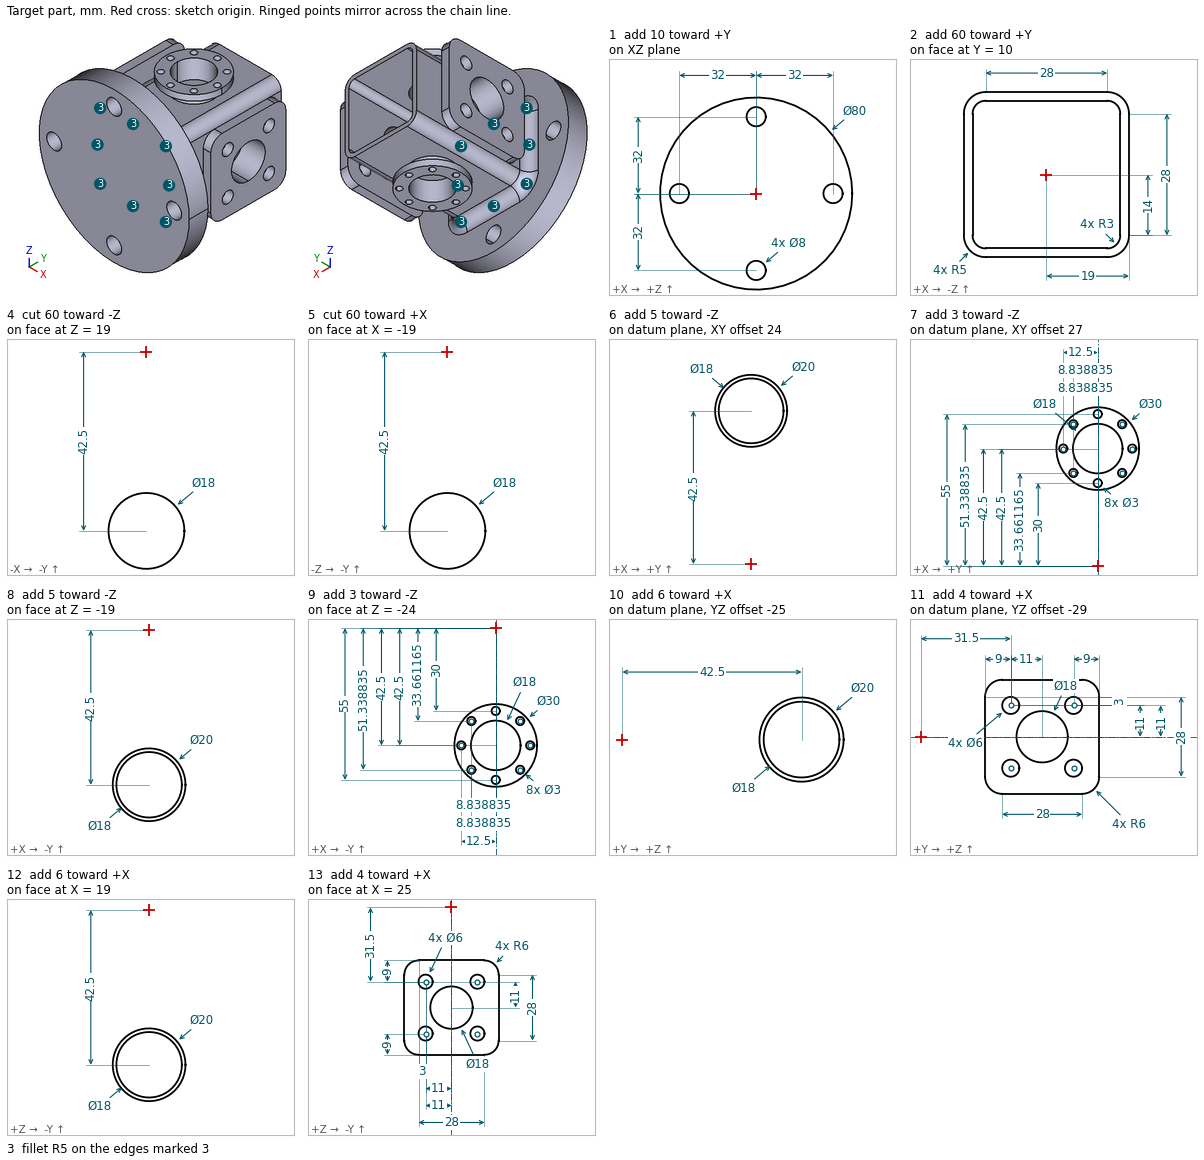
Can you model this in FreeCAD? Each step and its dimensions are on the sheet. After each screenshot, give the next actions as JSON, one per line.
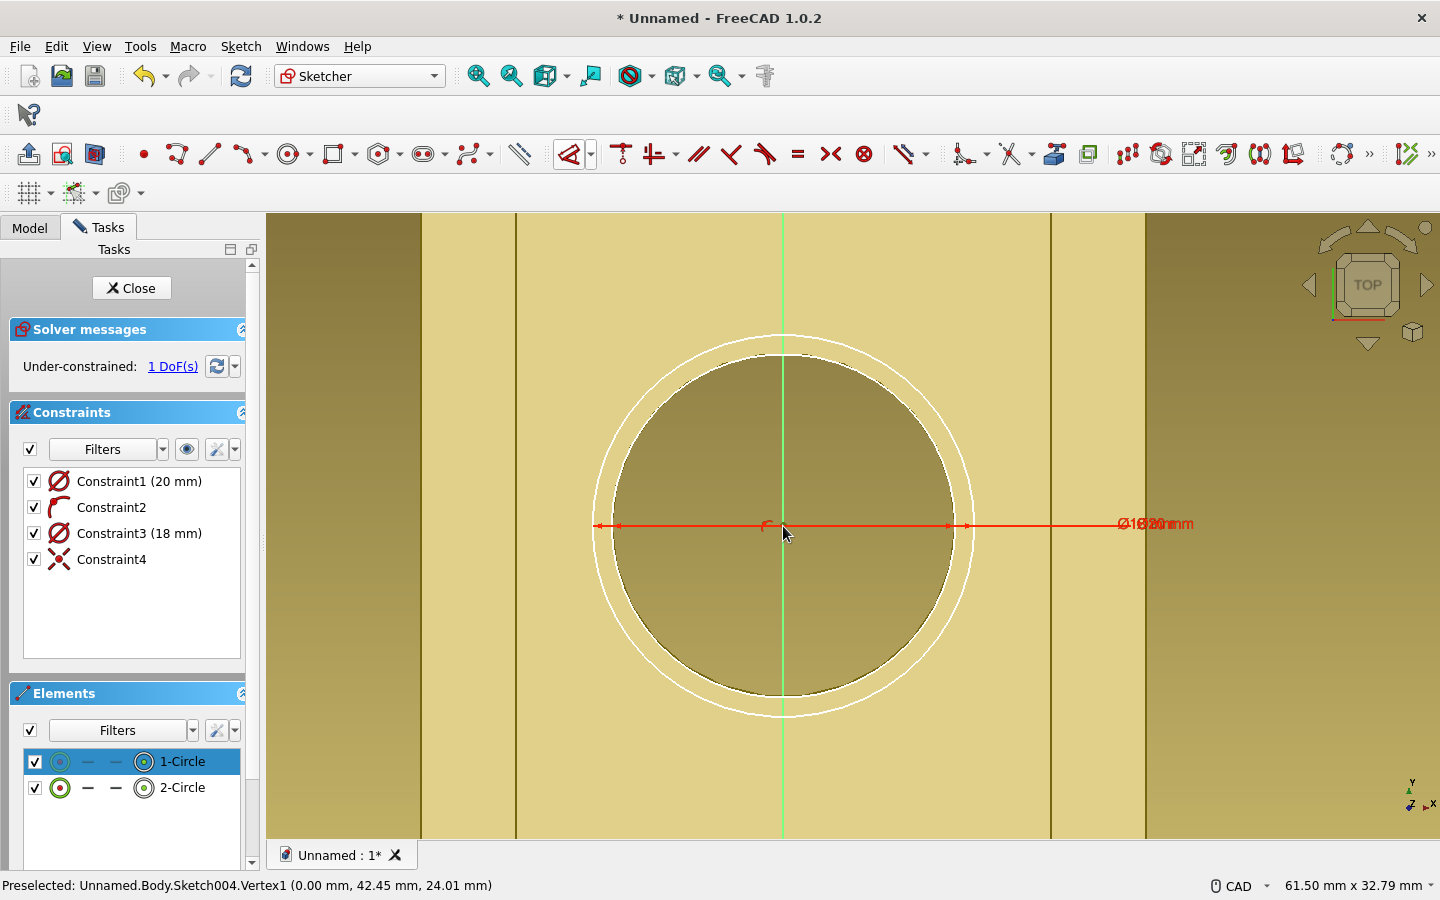
{"action": "key", "text": "i"}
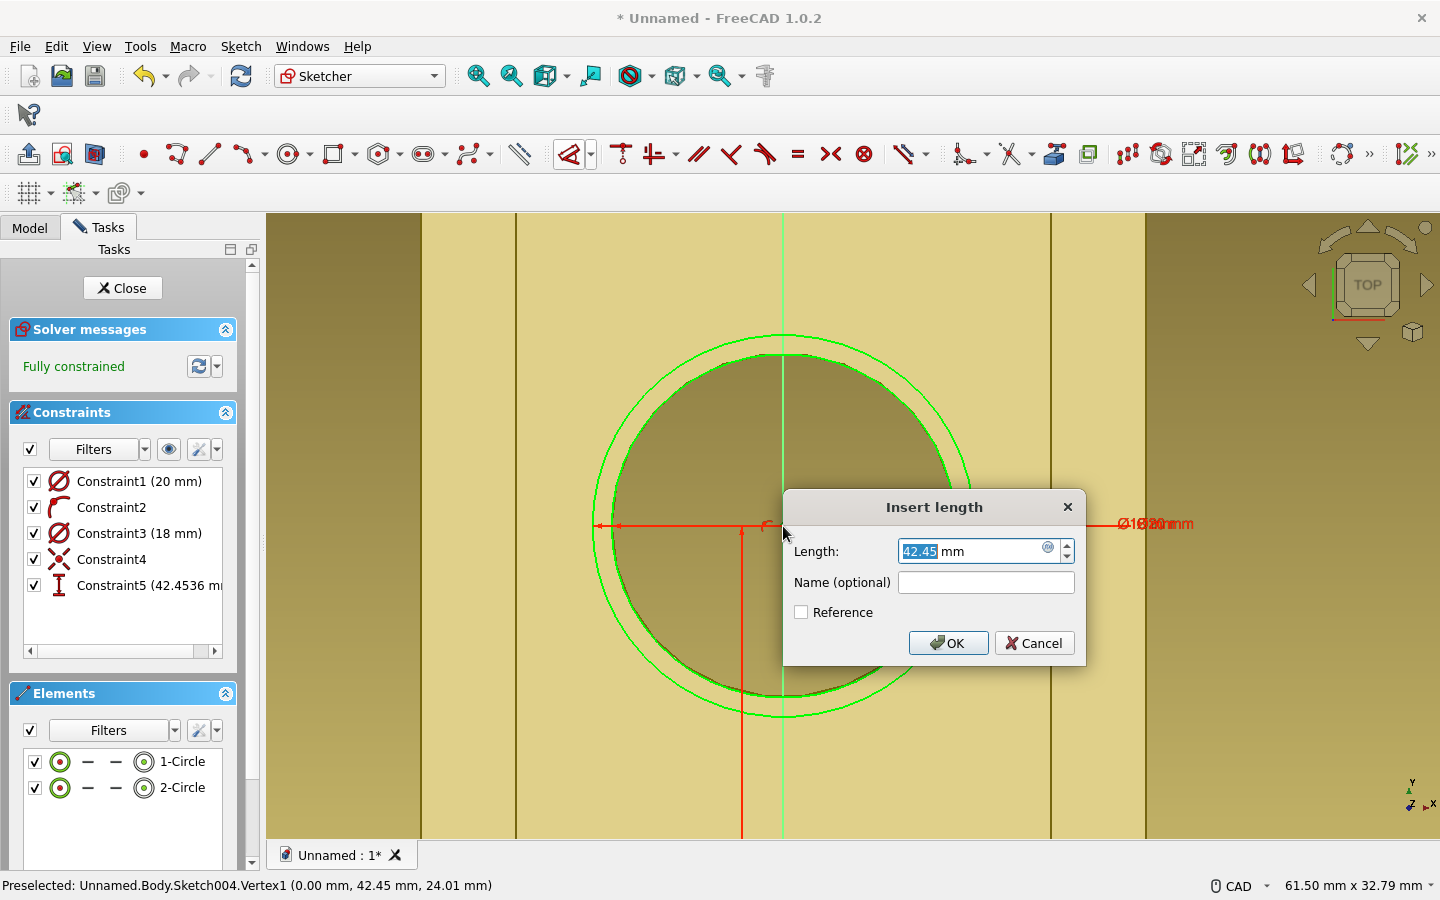
{"action": "type", "text": "42.5"}
{"action": "key", "text": "Return"}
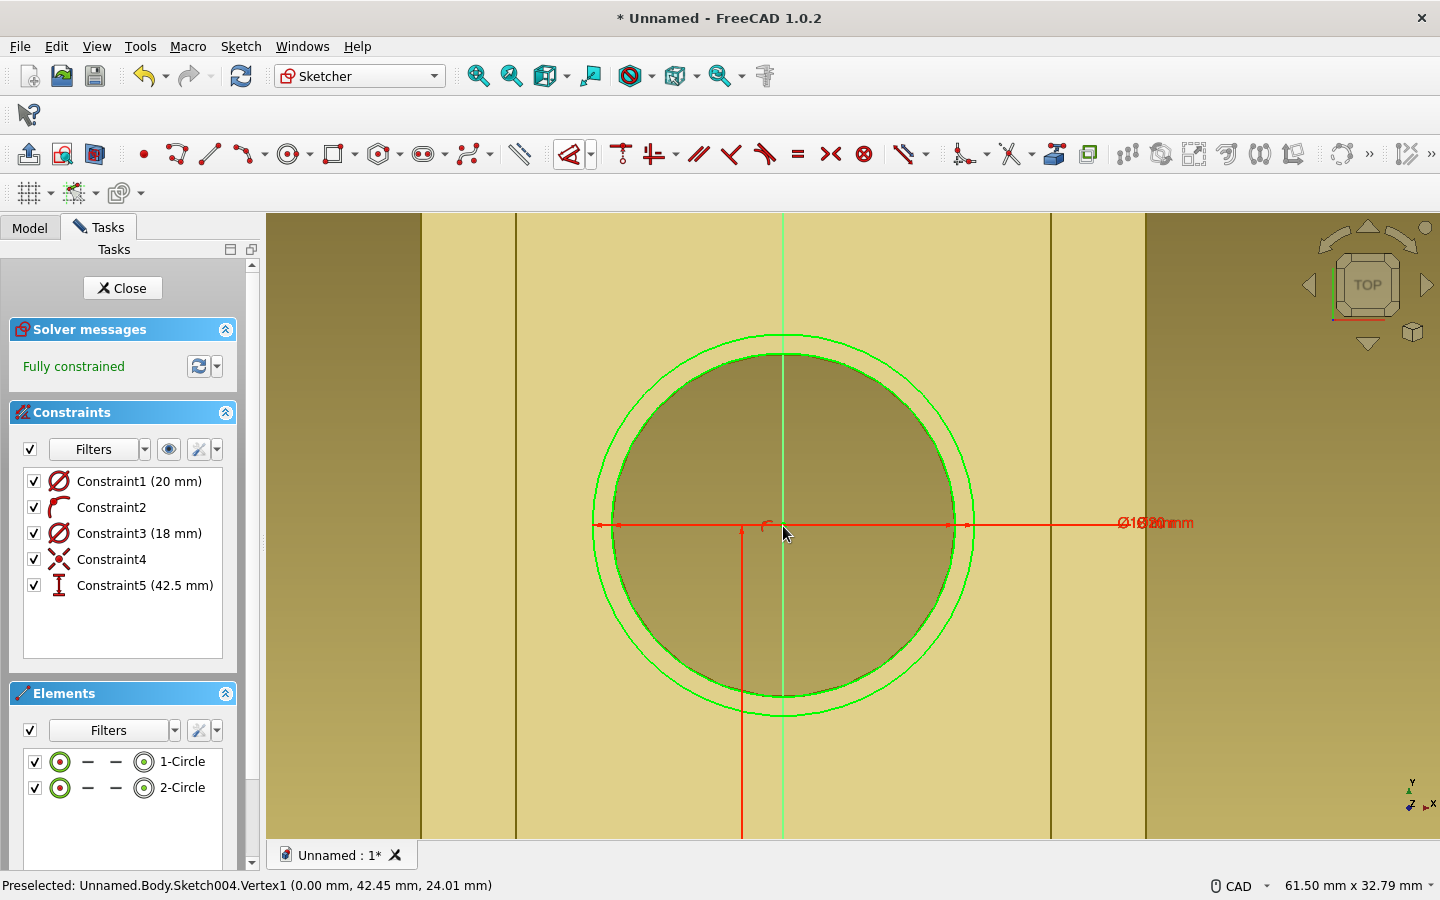
{"action": "left_click", "coordinate": [123, 288]}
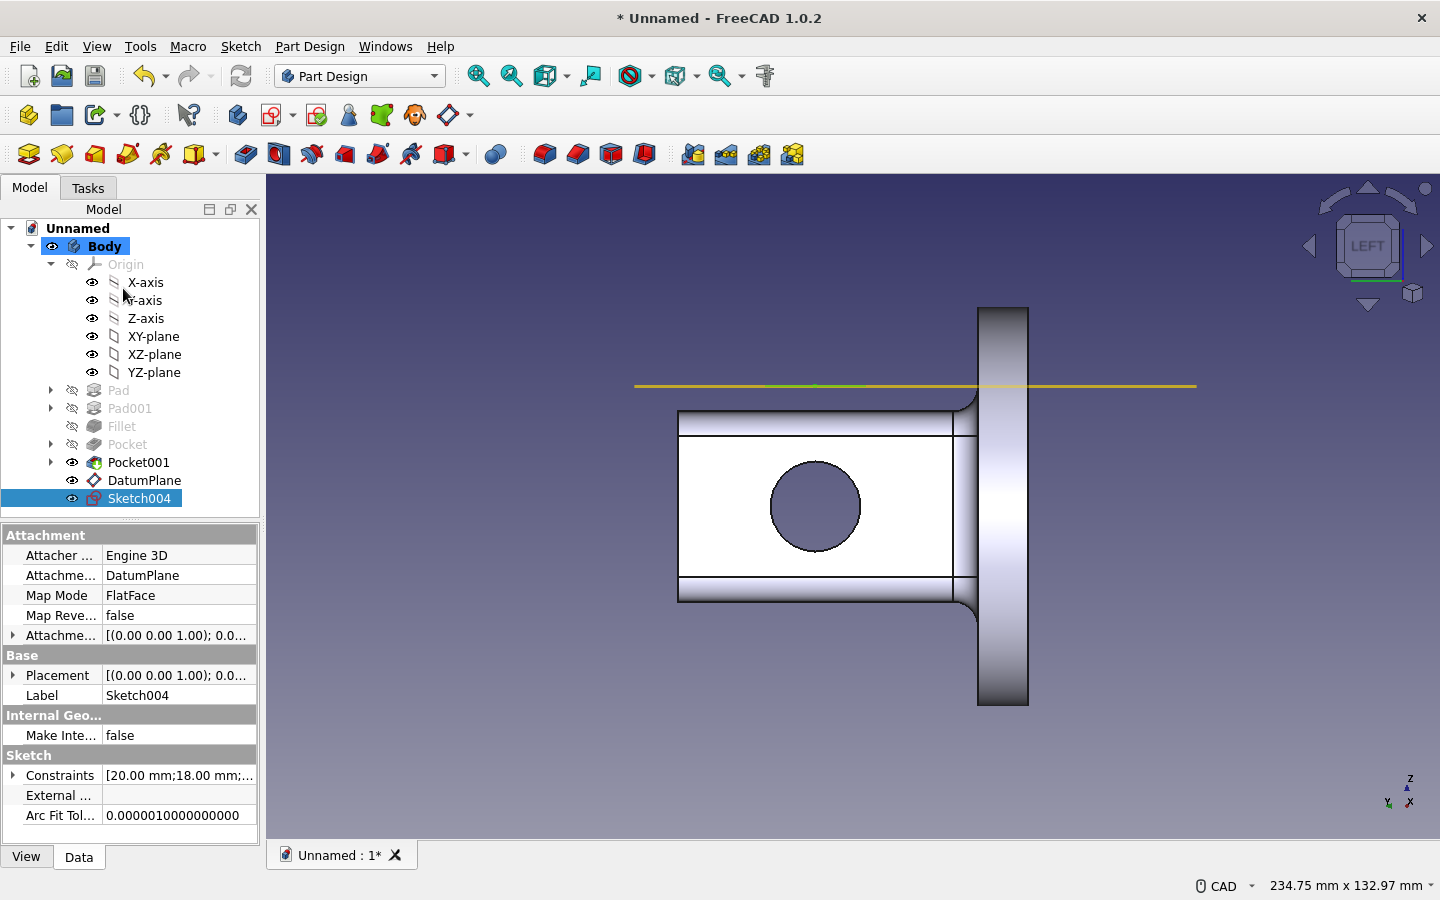
{"action": "left_click", "coordinate": [29, 154]}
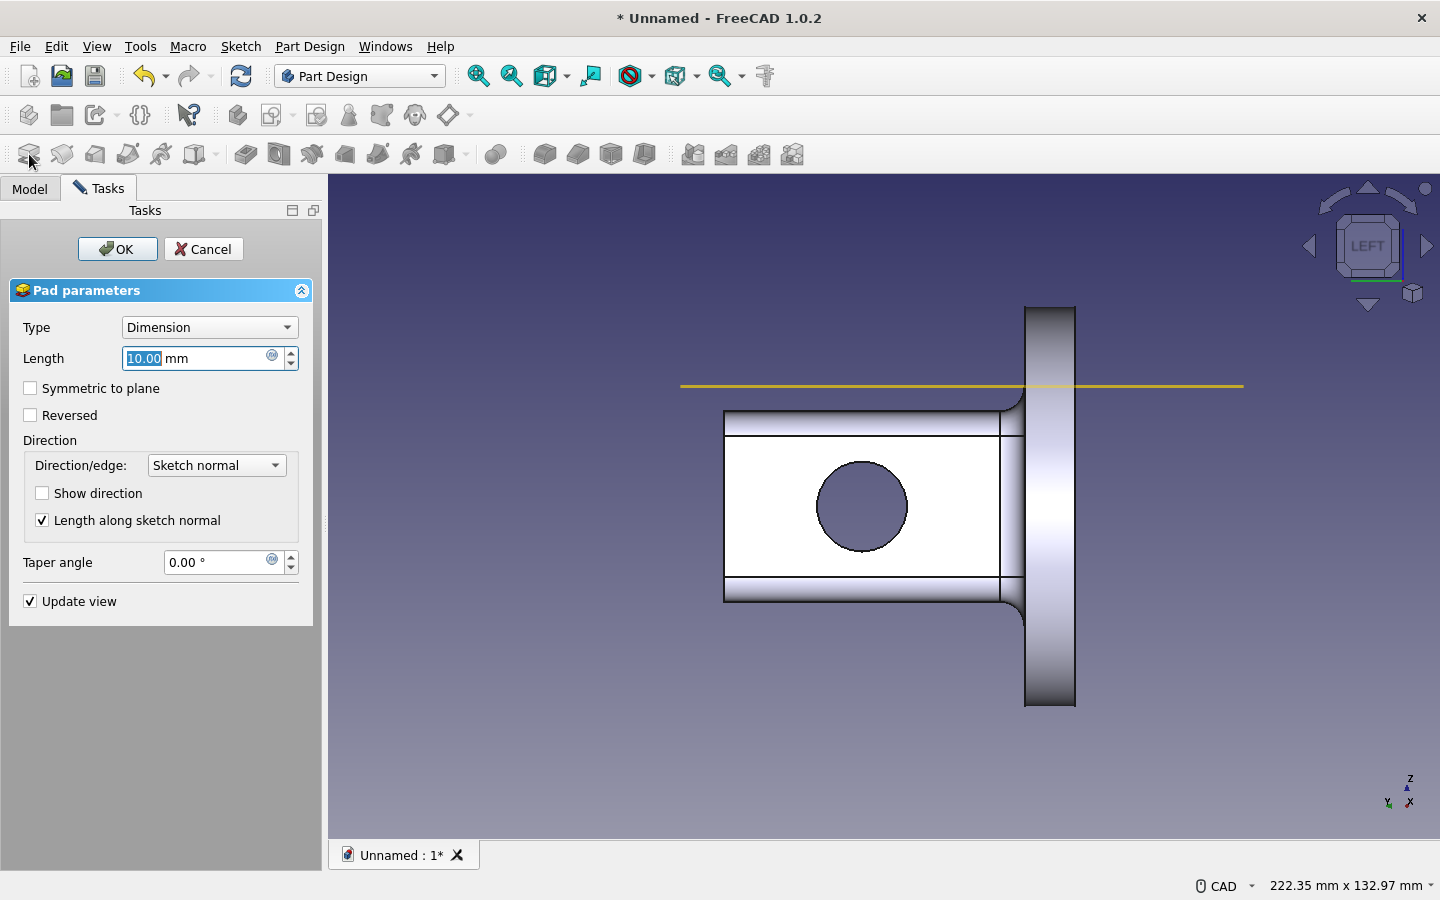
{"action": "type", "text": "5"}
{"action": "key", "text": "Tab"}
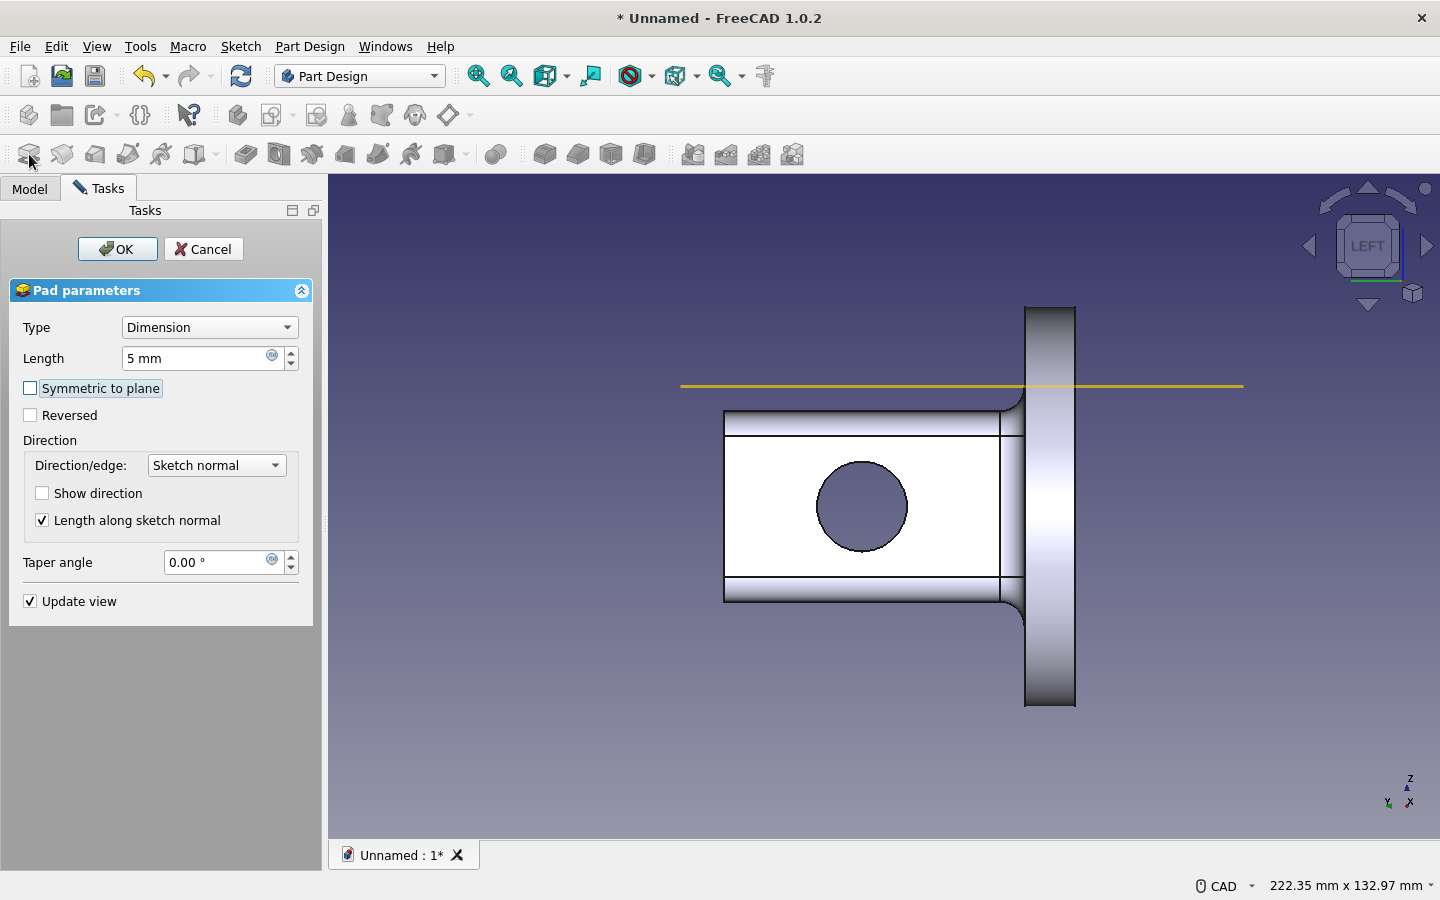
{"action": "left_click", "coordinate": [31, 415]}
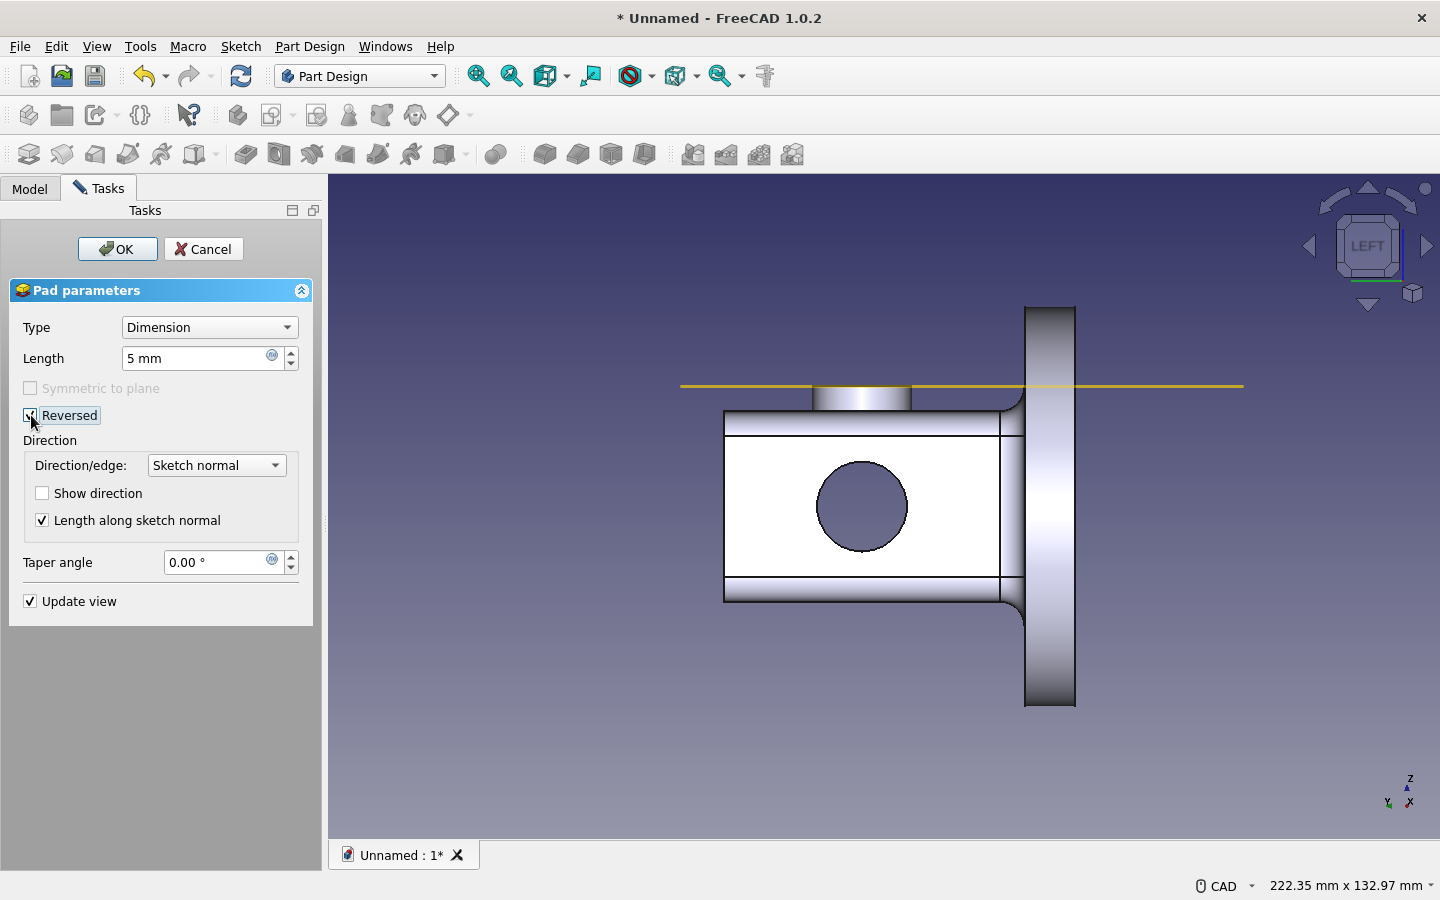
{"action": "left_click", "coordinate": [118, 249]}